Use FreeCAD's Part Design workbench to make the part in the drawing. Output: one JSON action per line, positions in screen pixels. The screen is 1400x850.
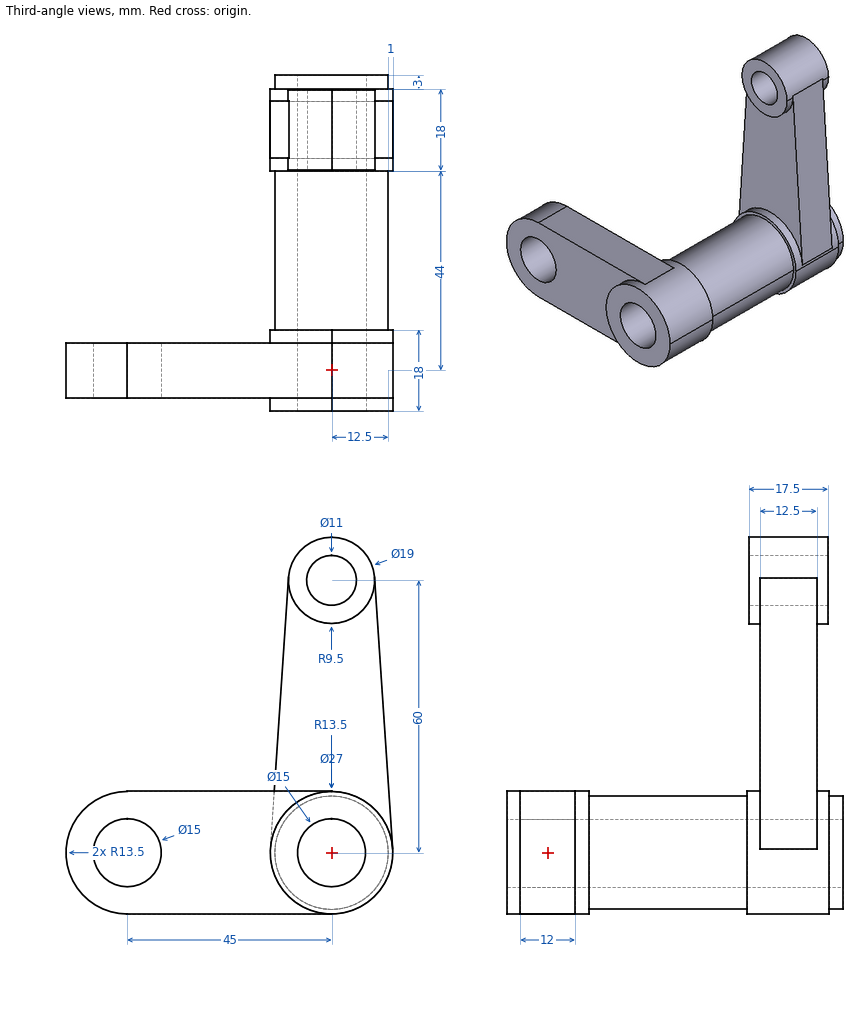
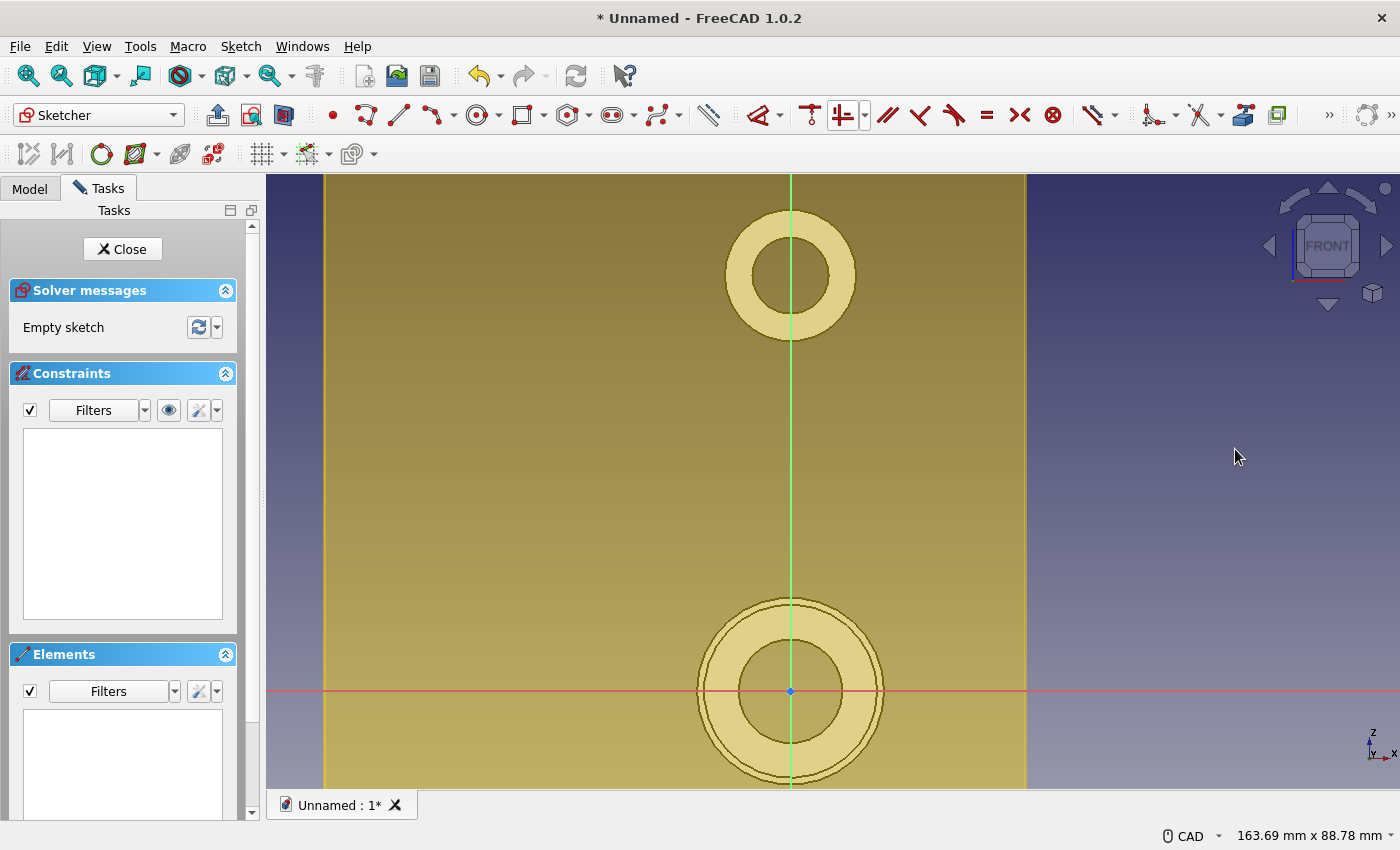
{"action": "key", "text": "g l"}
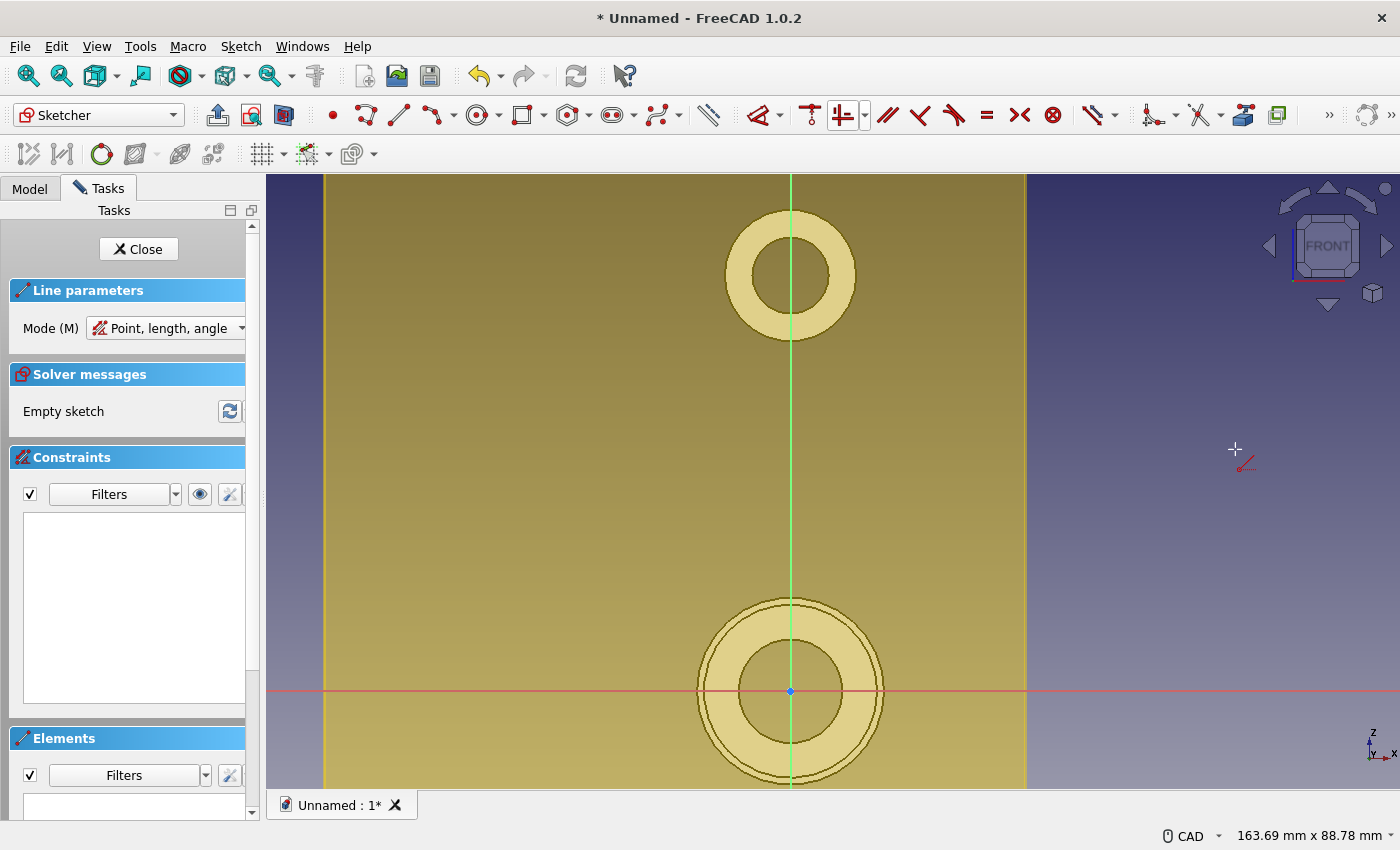
{"action": "left_click", "coordinate": [856, 271]}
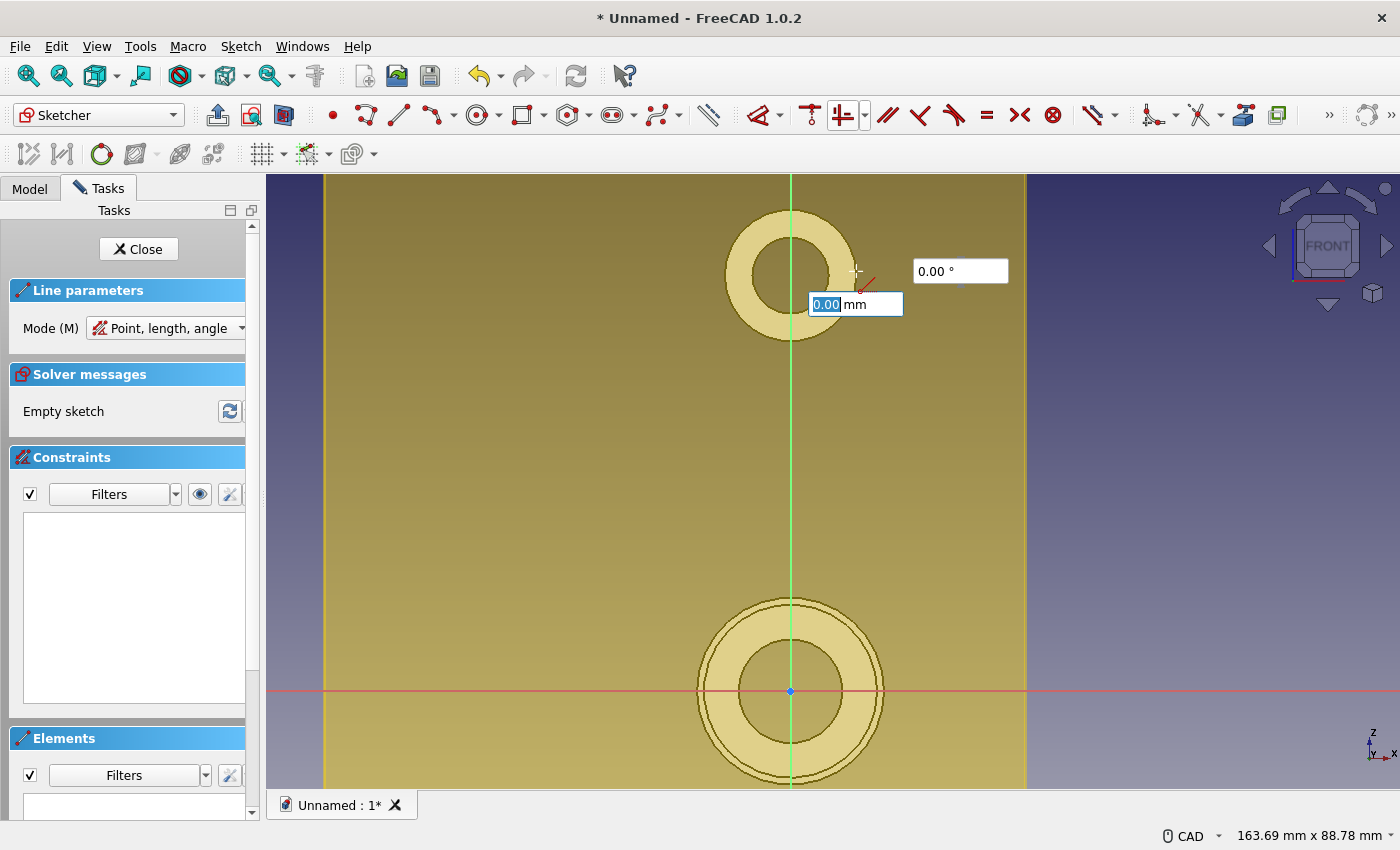
{"action": "scroll", "coordinate": [884, 685], "scroll_direction": "up", "scroll_amount": 5}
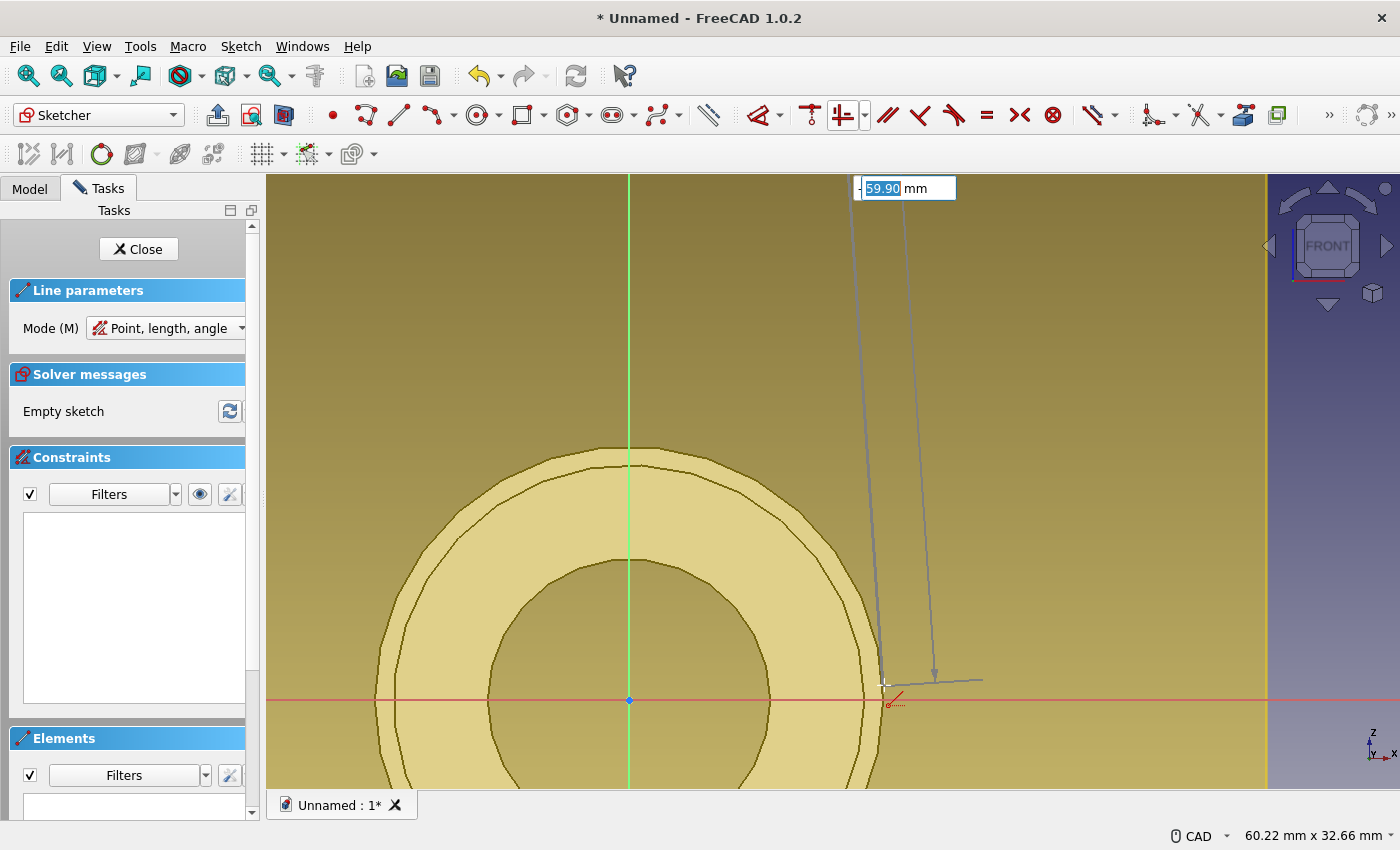
{"action": "left_click", "coordinate": [883, 684]}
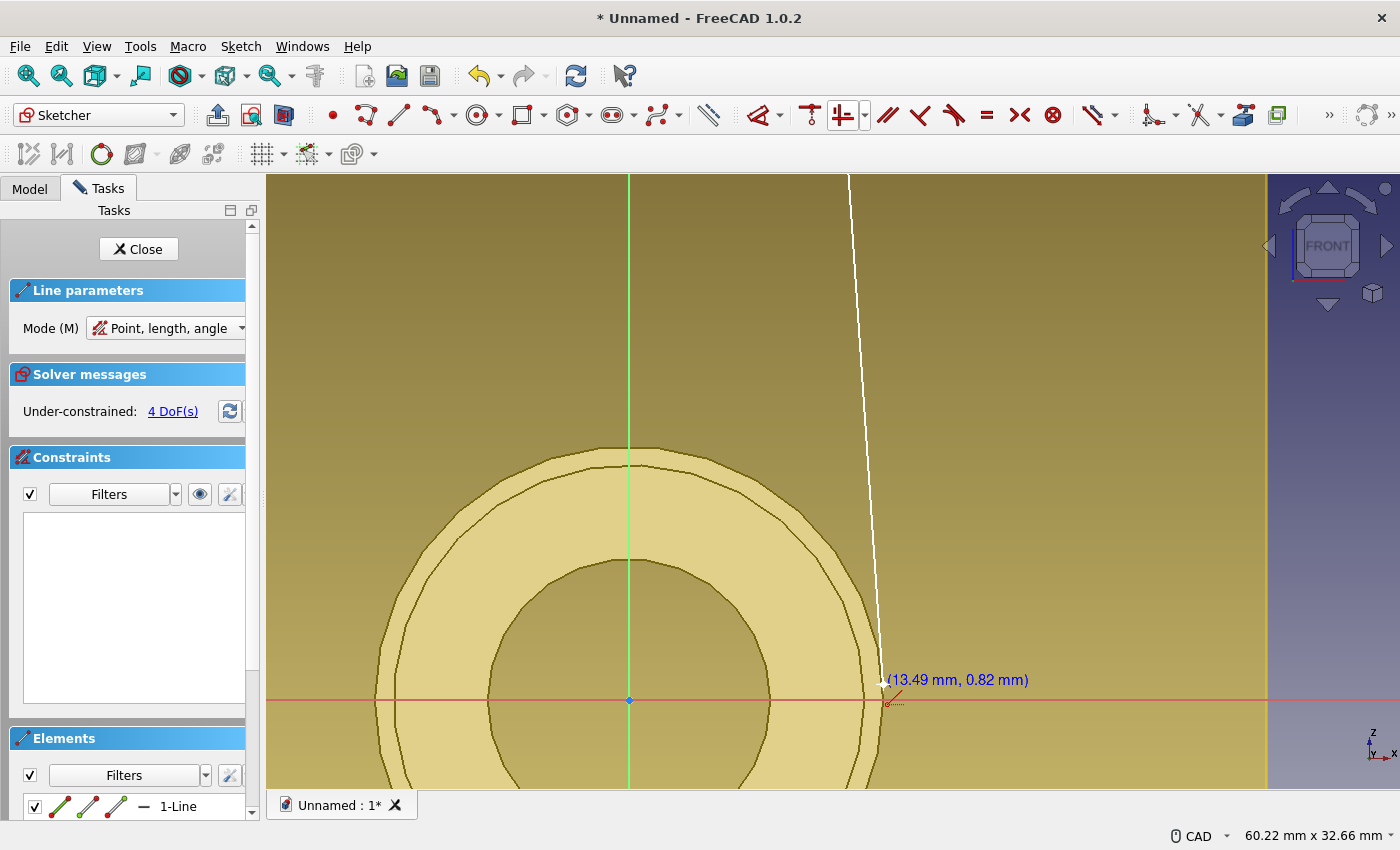
{"action": "left_click", "coordinate": [375, 684]}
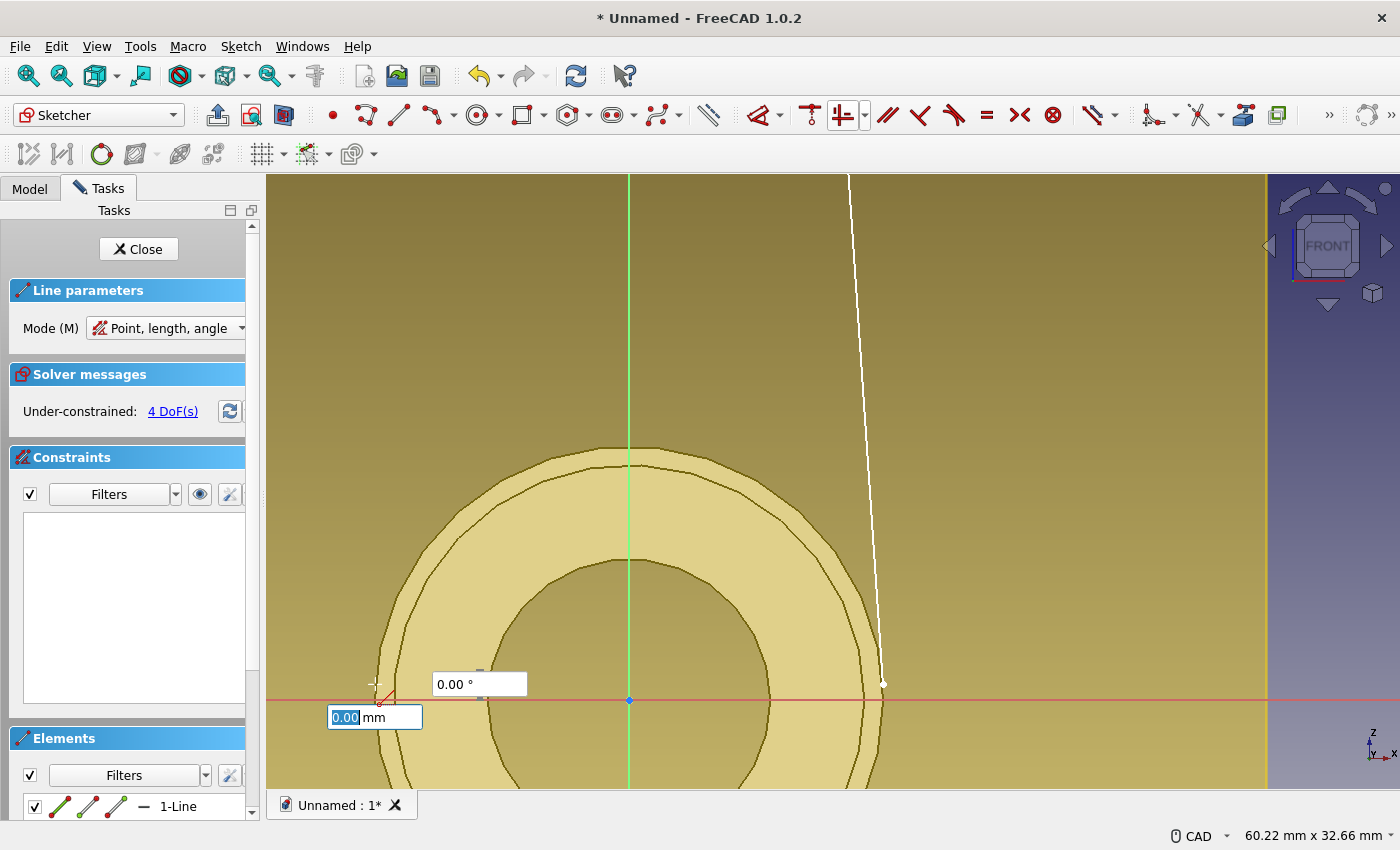
{"action": "scroll", "coordinate": [843, 686], "scroll_direction": "down", "scroll_amount": 5}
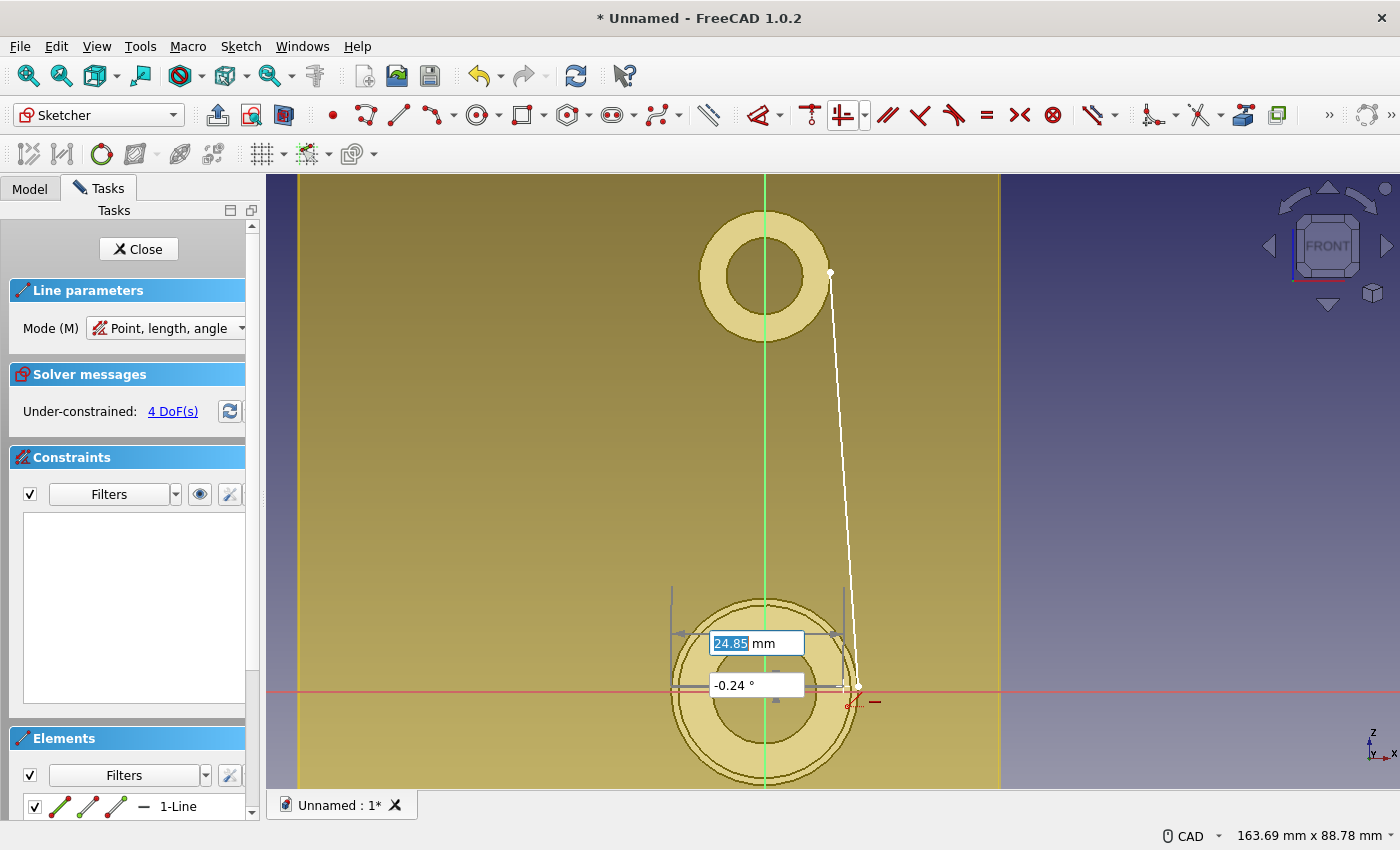
{"action": "left_click", "coordinate": [699, 272]}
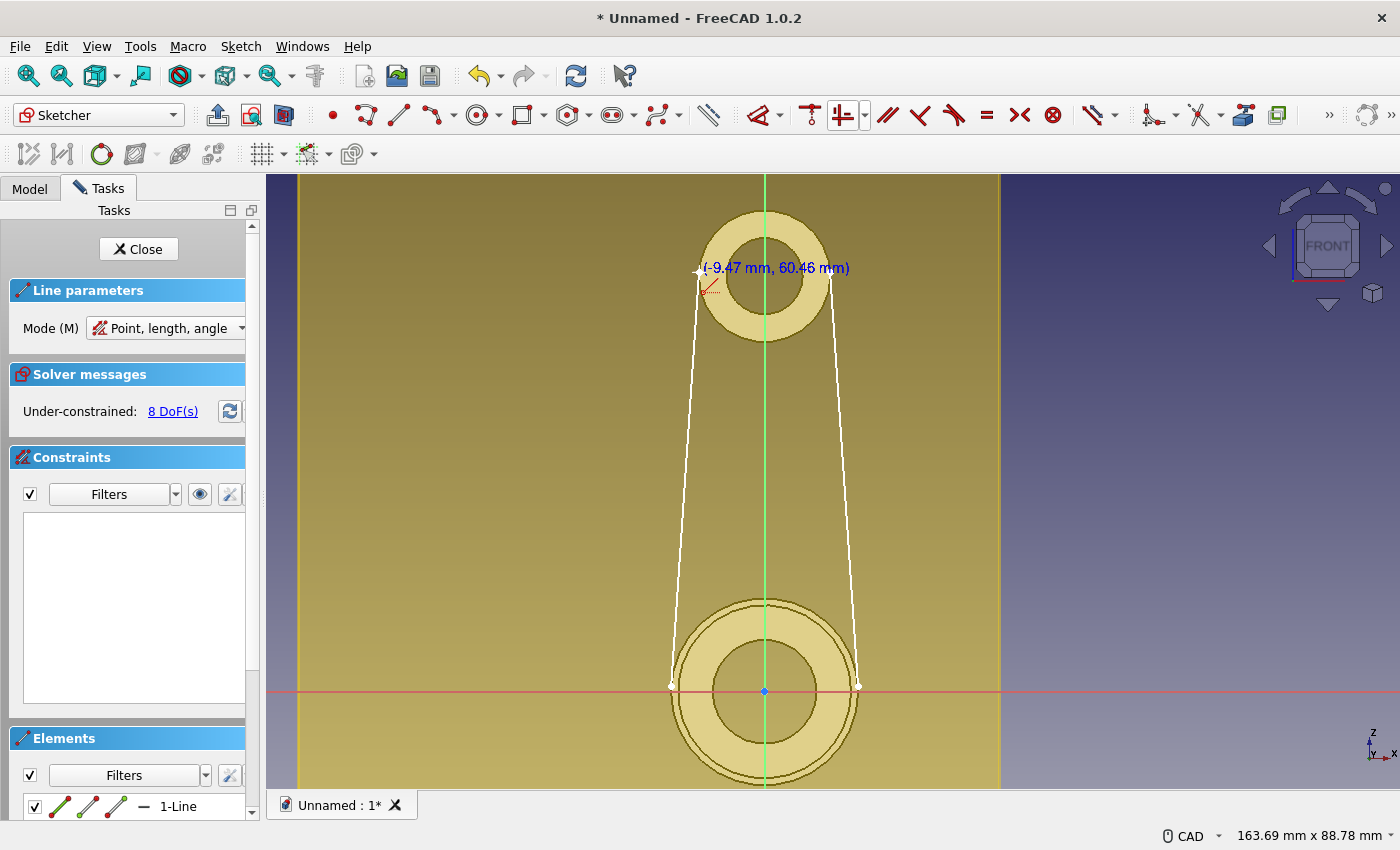
{"action": "key", "text": "g 3 a"}